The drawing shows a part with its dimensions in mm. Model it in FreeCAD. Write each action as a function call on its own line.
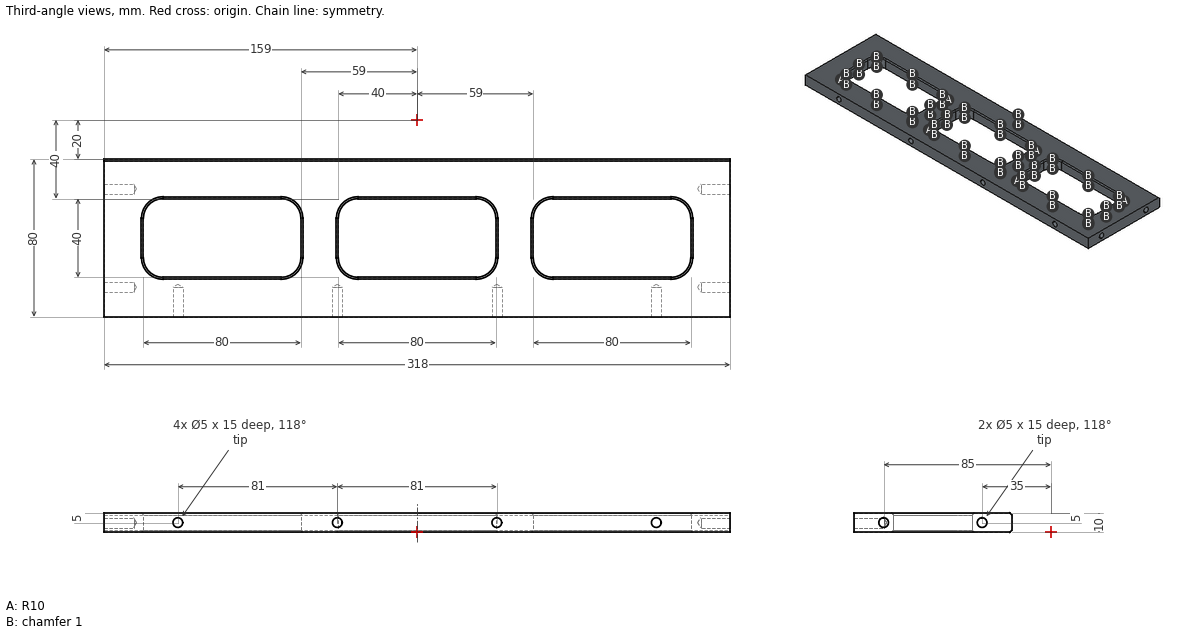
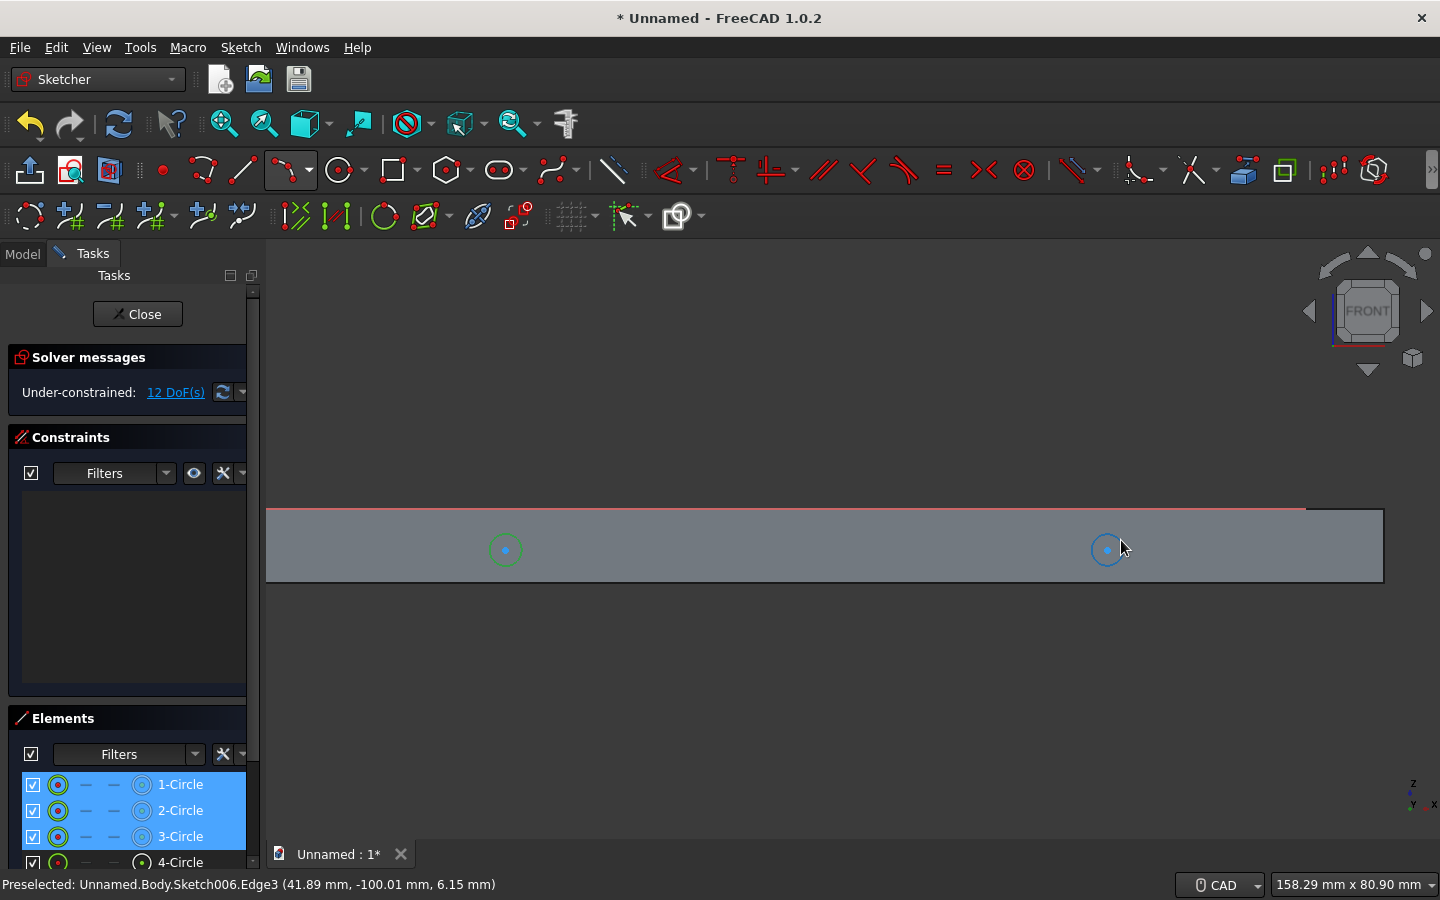
click(1118, 539)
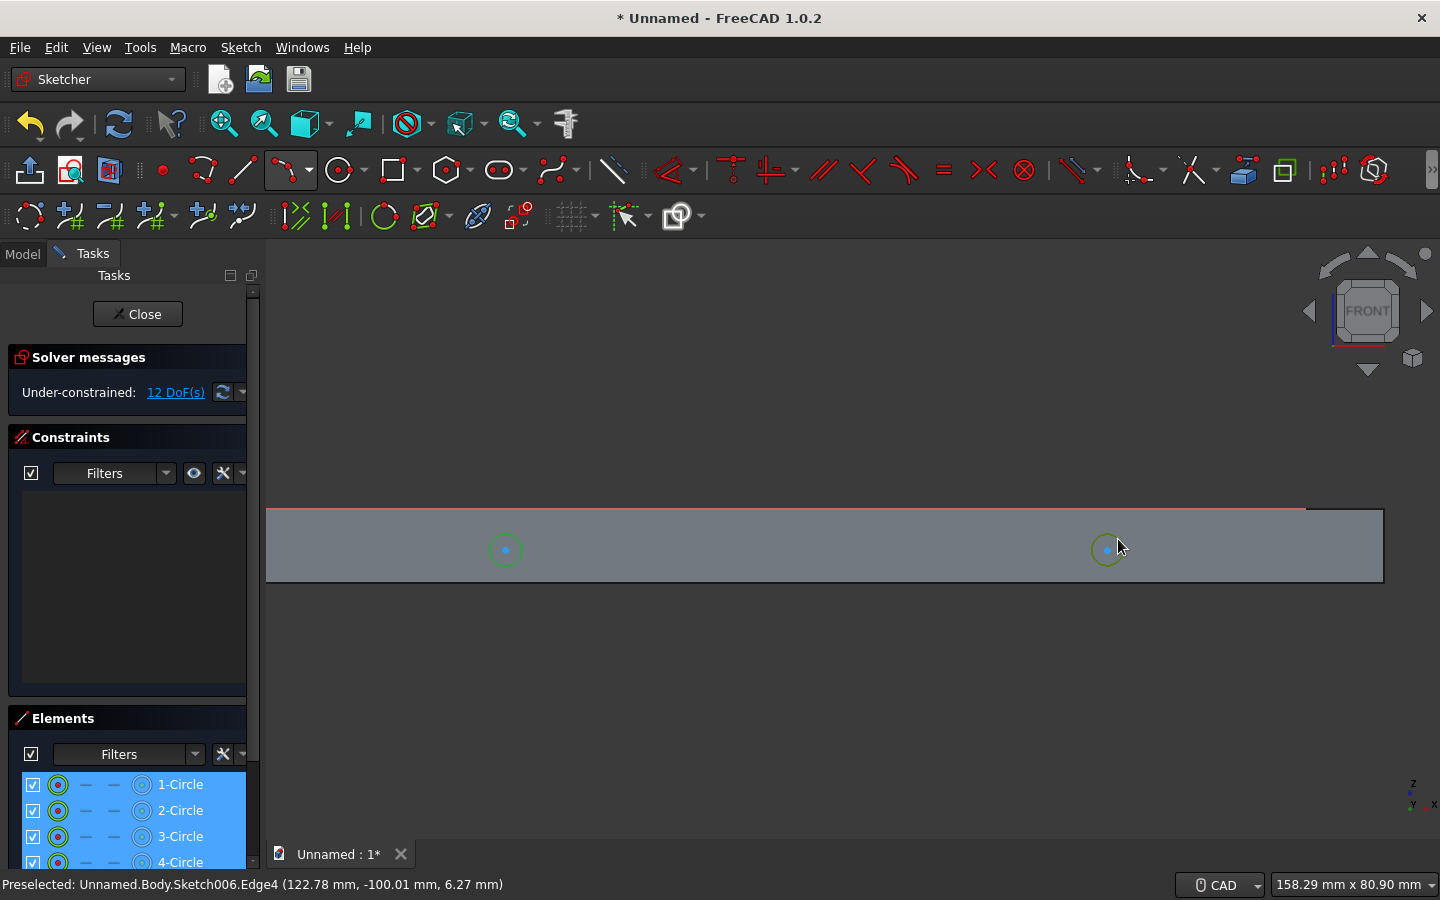
key(e)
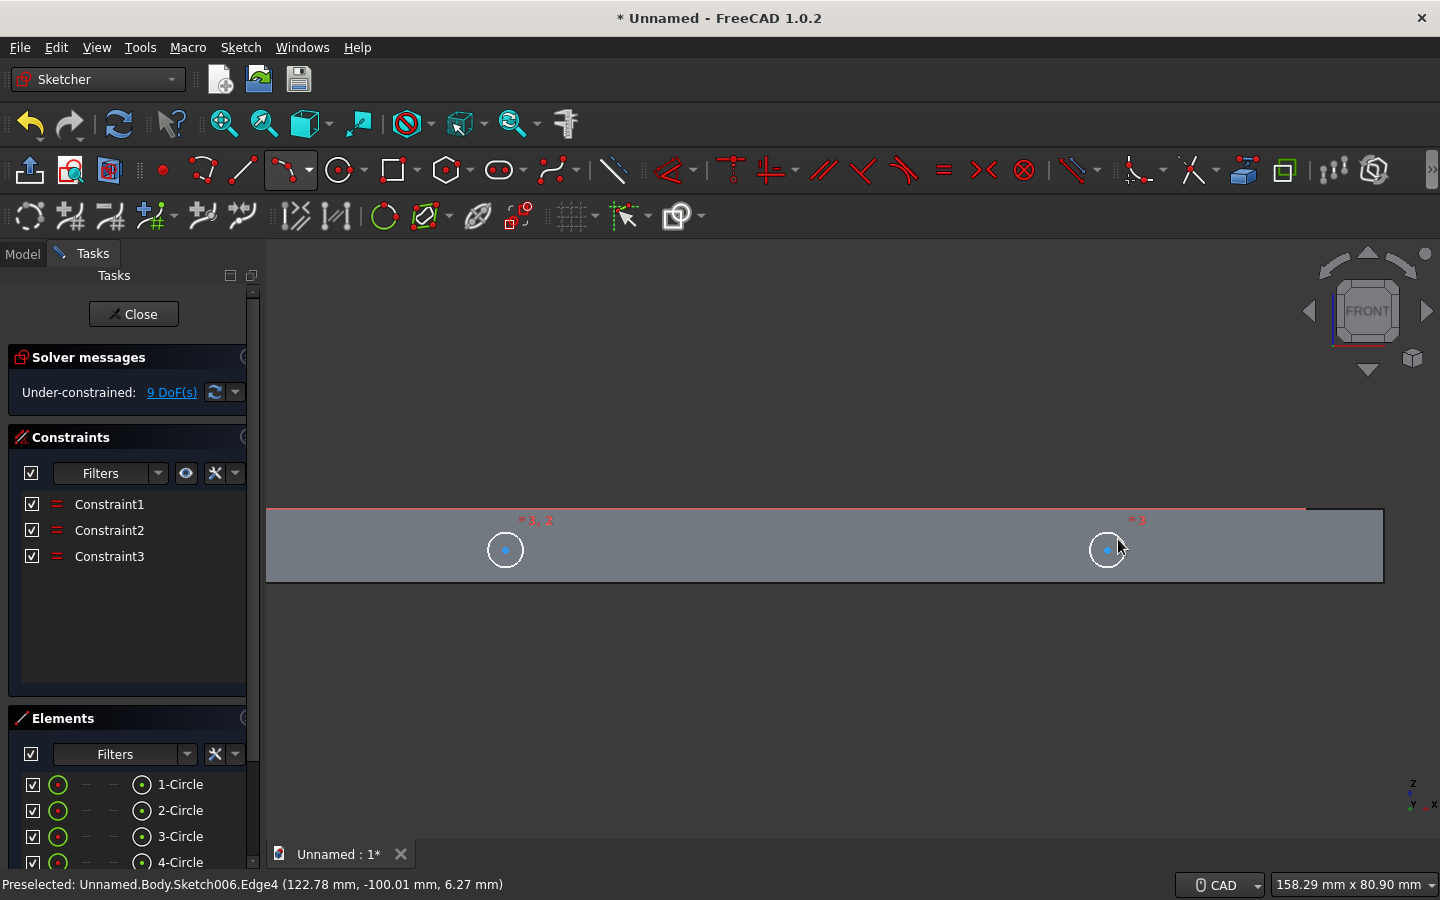
scroll(1122, 540, down, 5)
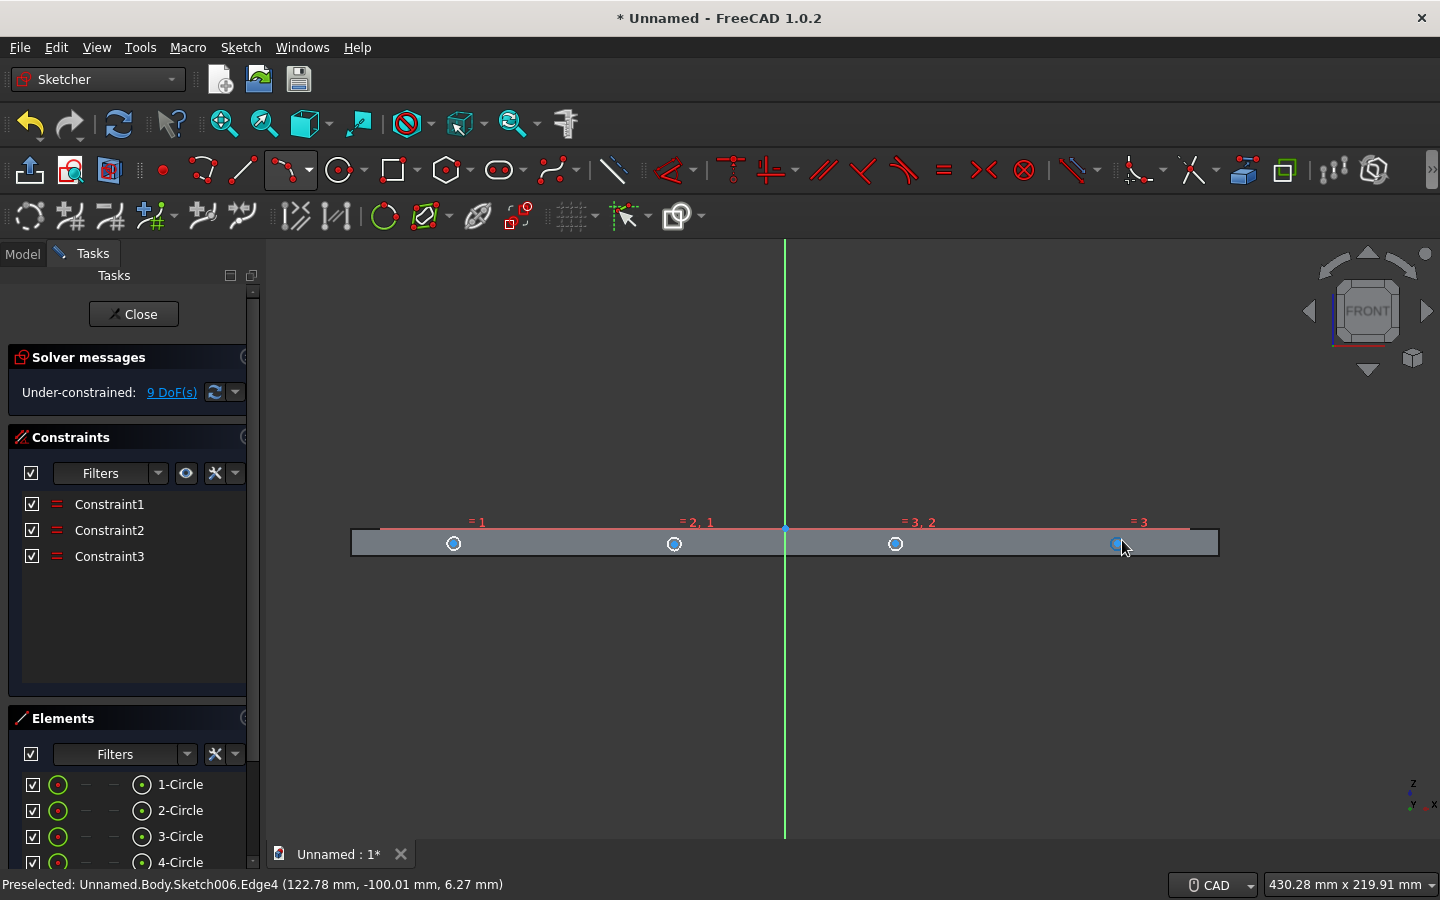
click(674, 544)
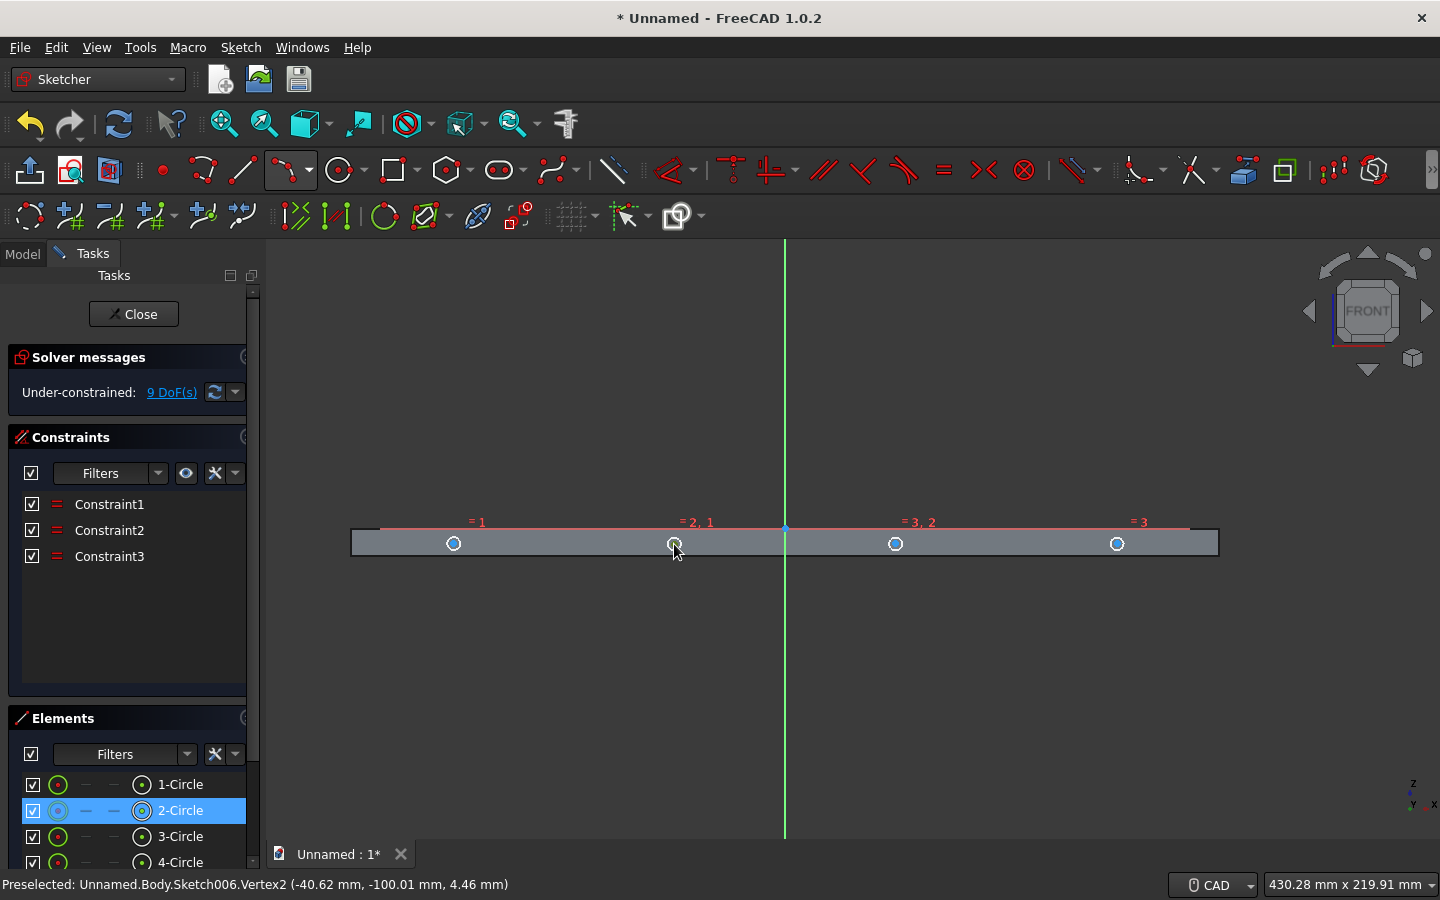
click(896, 544)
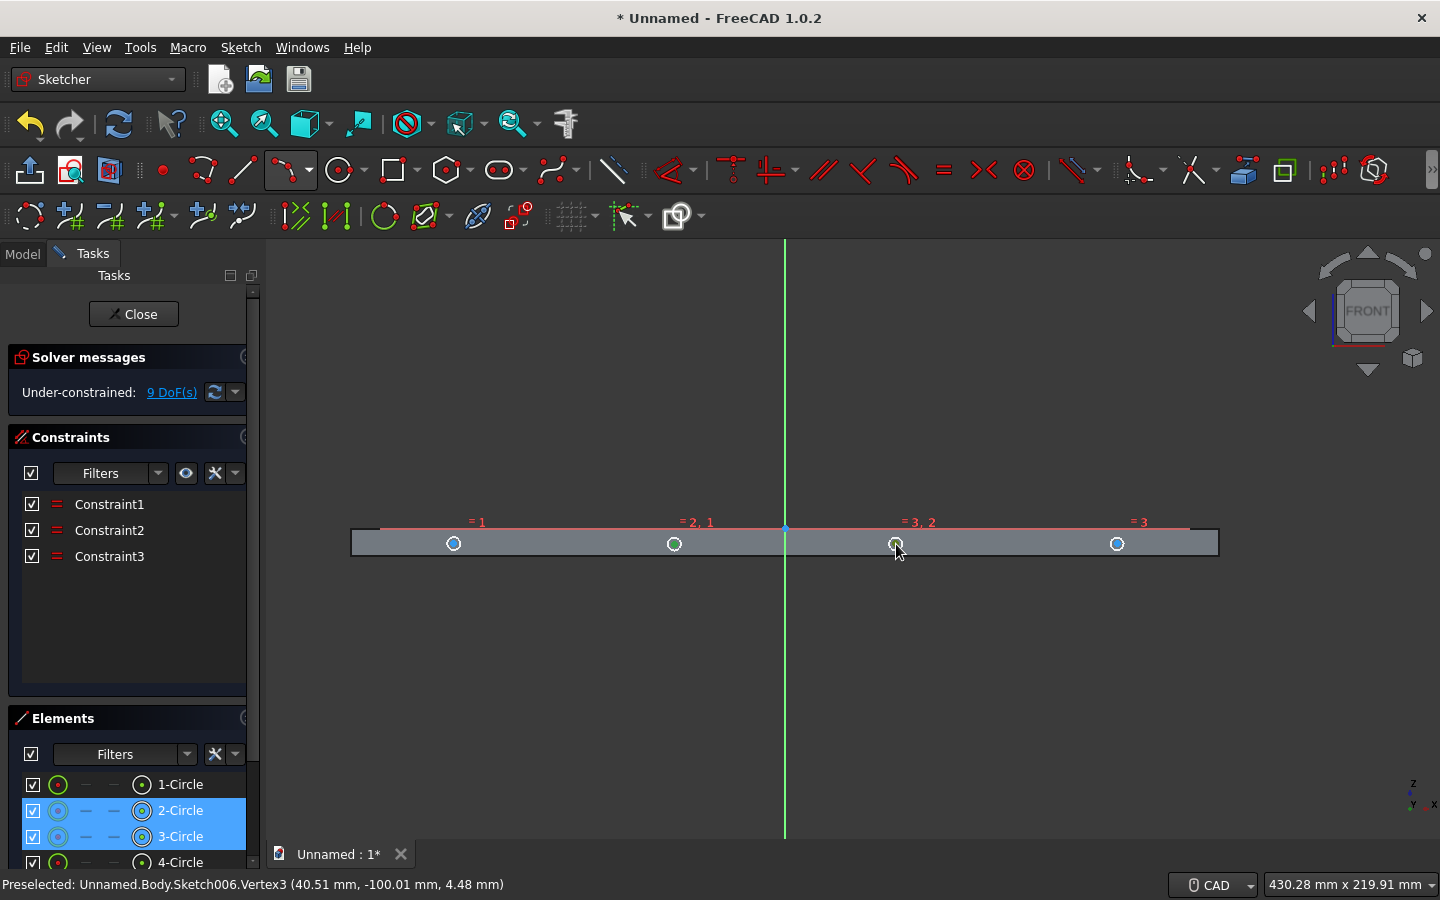
click(785, 772)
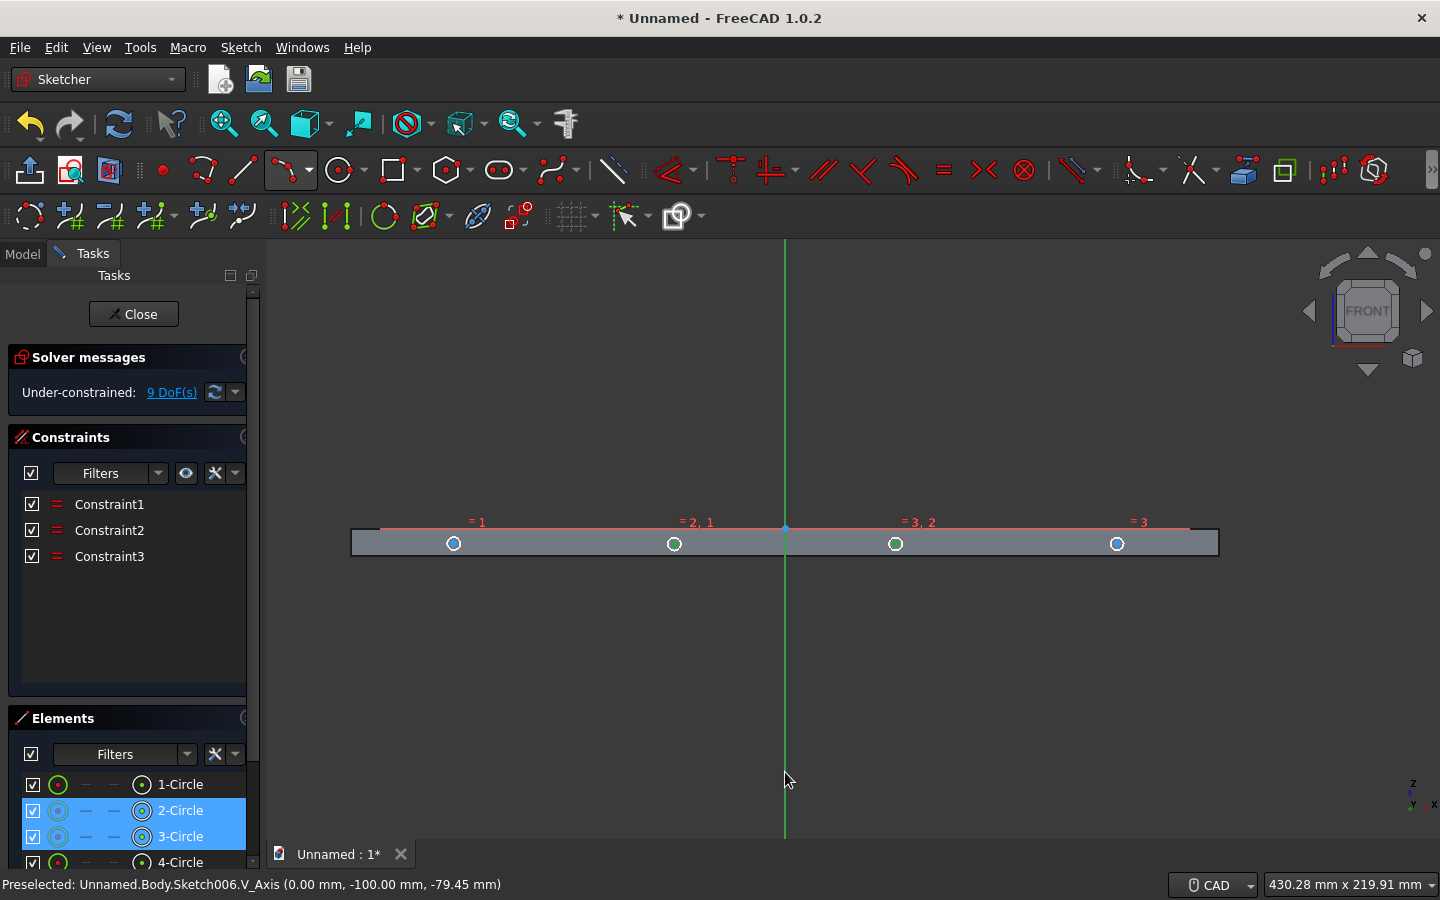
click(984, 170)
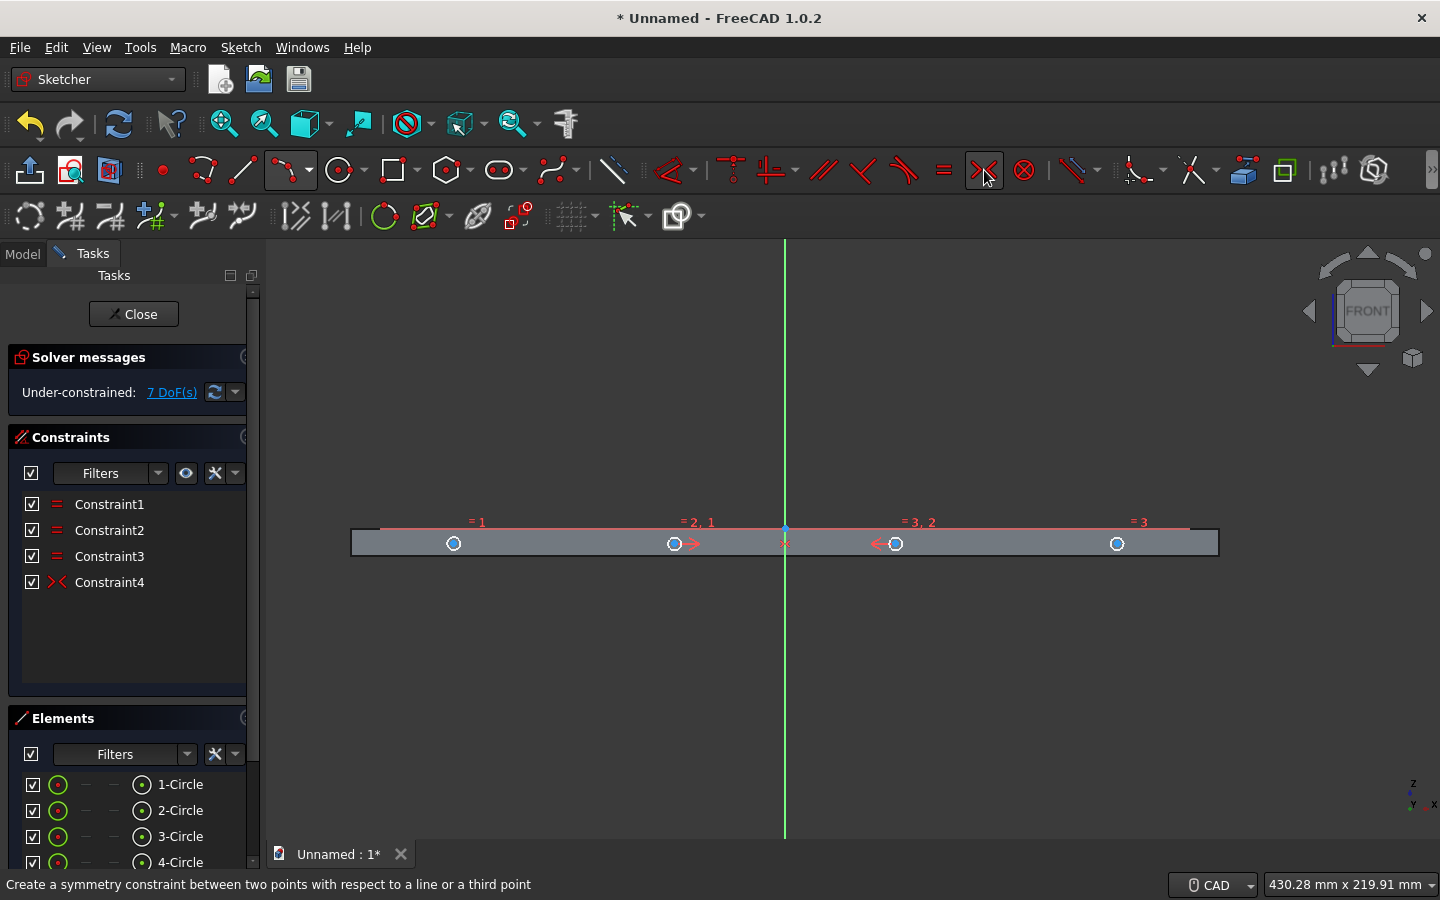
click(454, 544)